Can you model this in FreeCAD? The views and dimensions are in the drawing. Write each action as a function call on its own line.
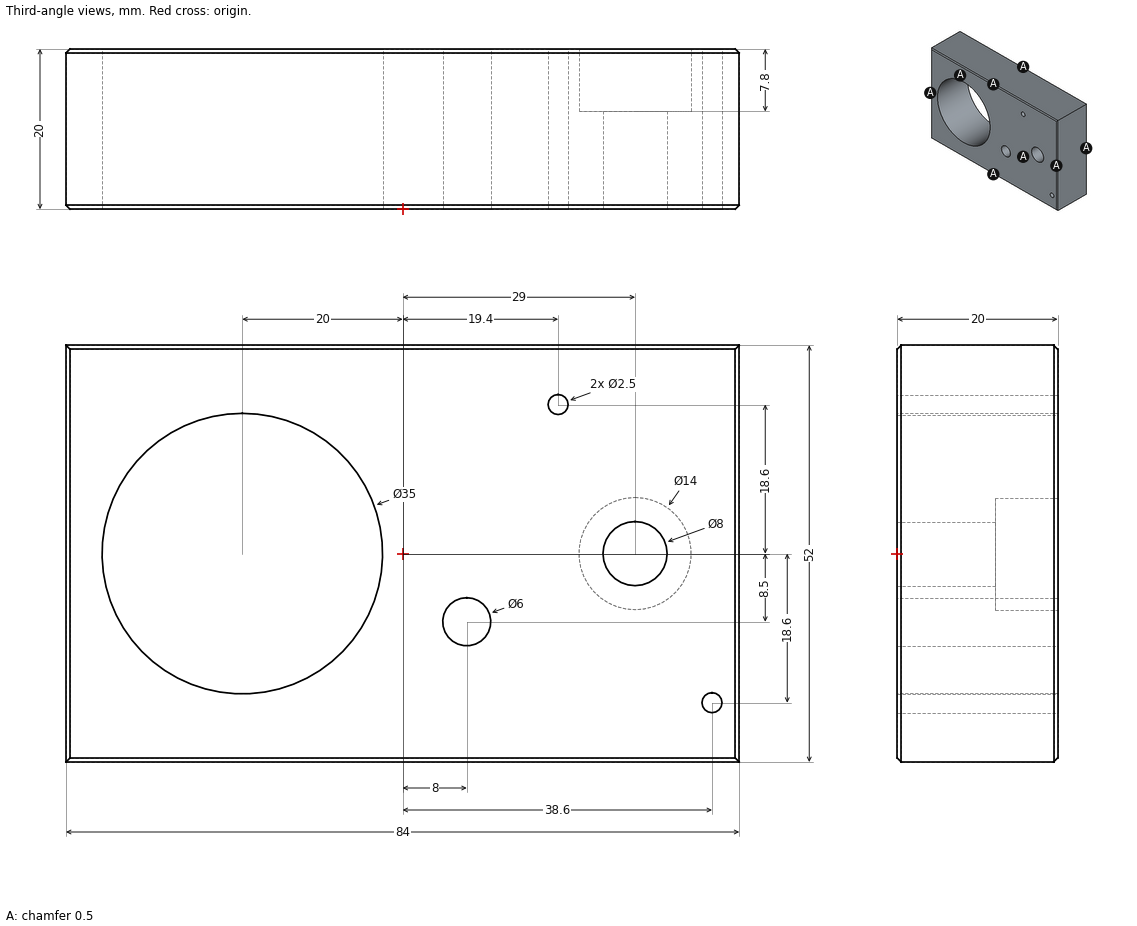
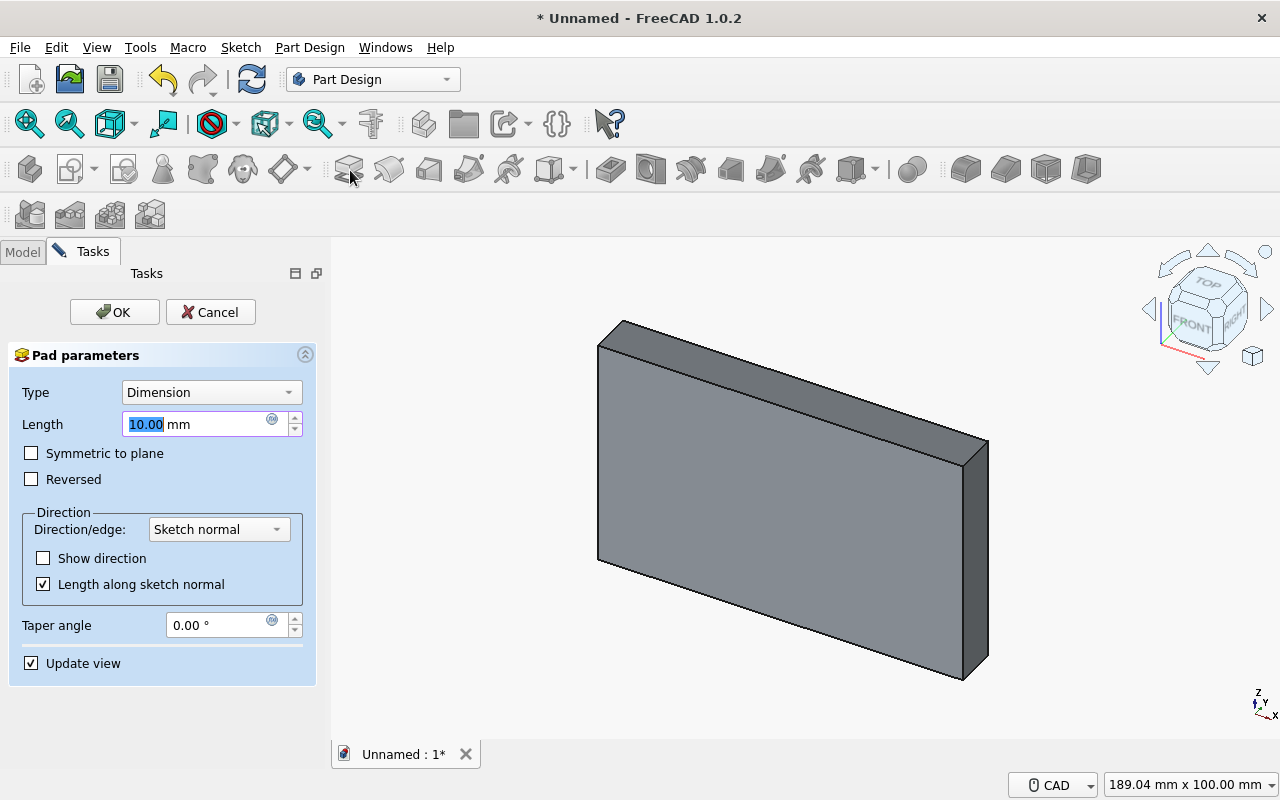
text(20)
key(Tab)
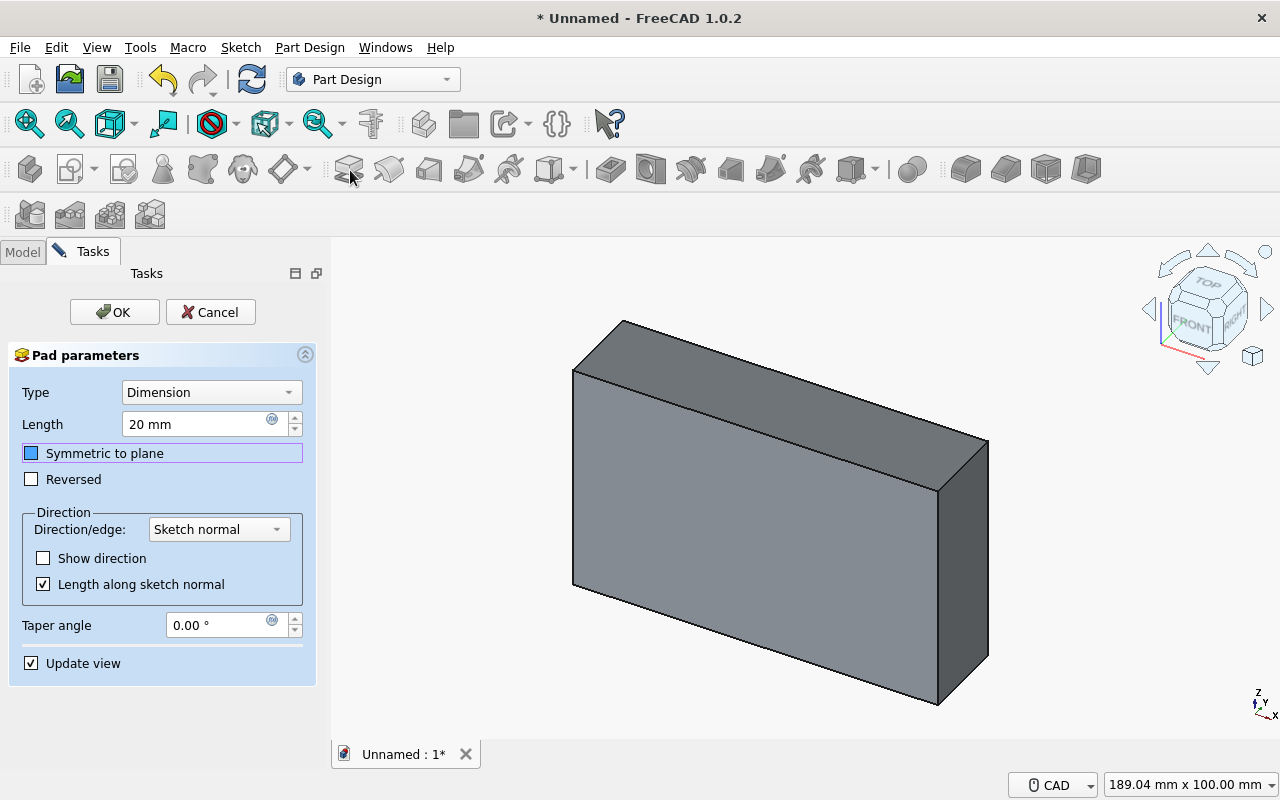
click(30, 479)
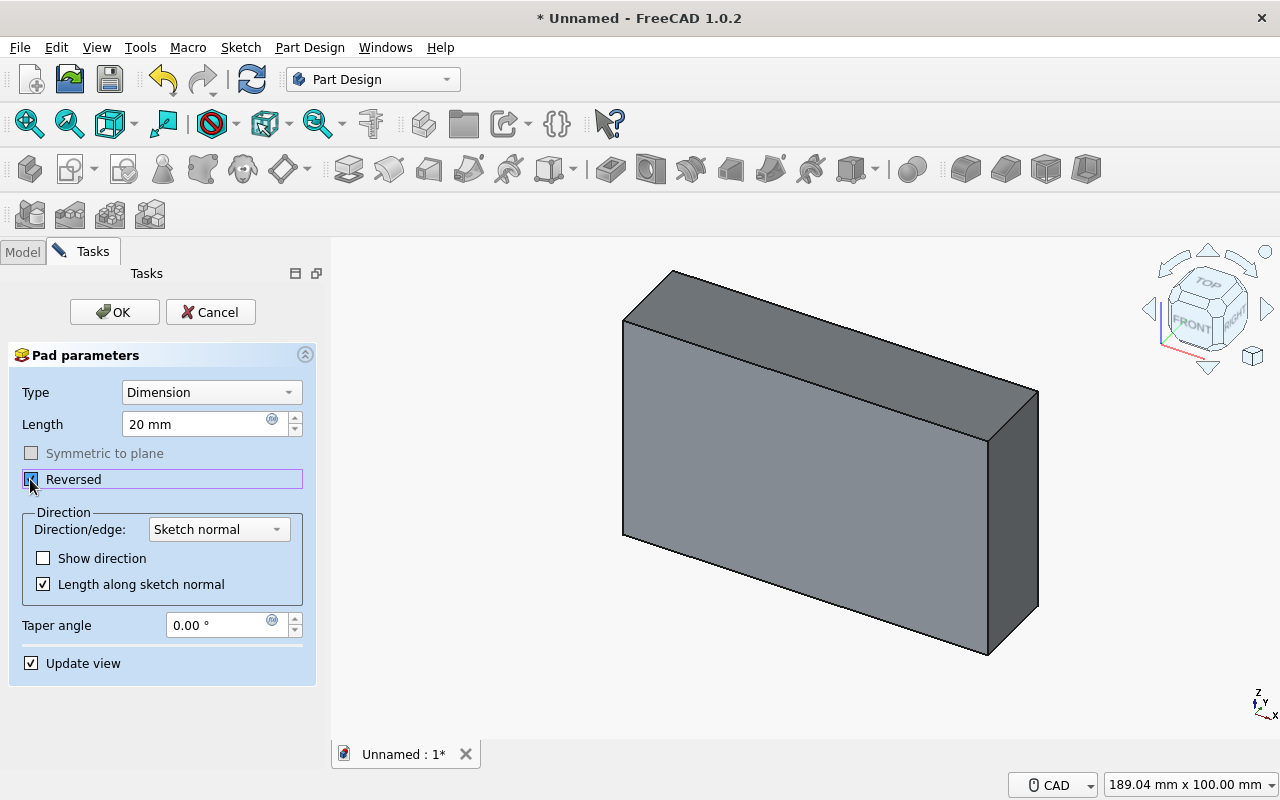
click(115, 312)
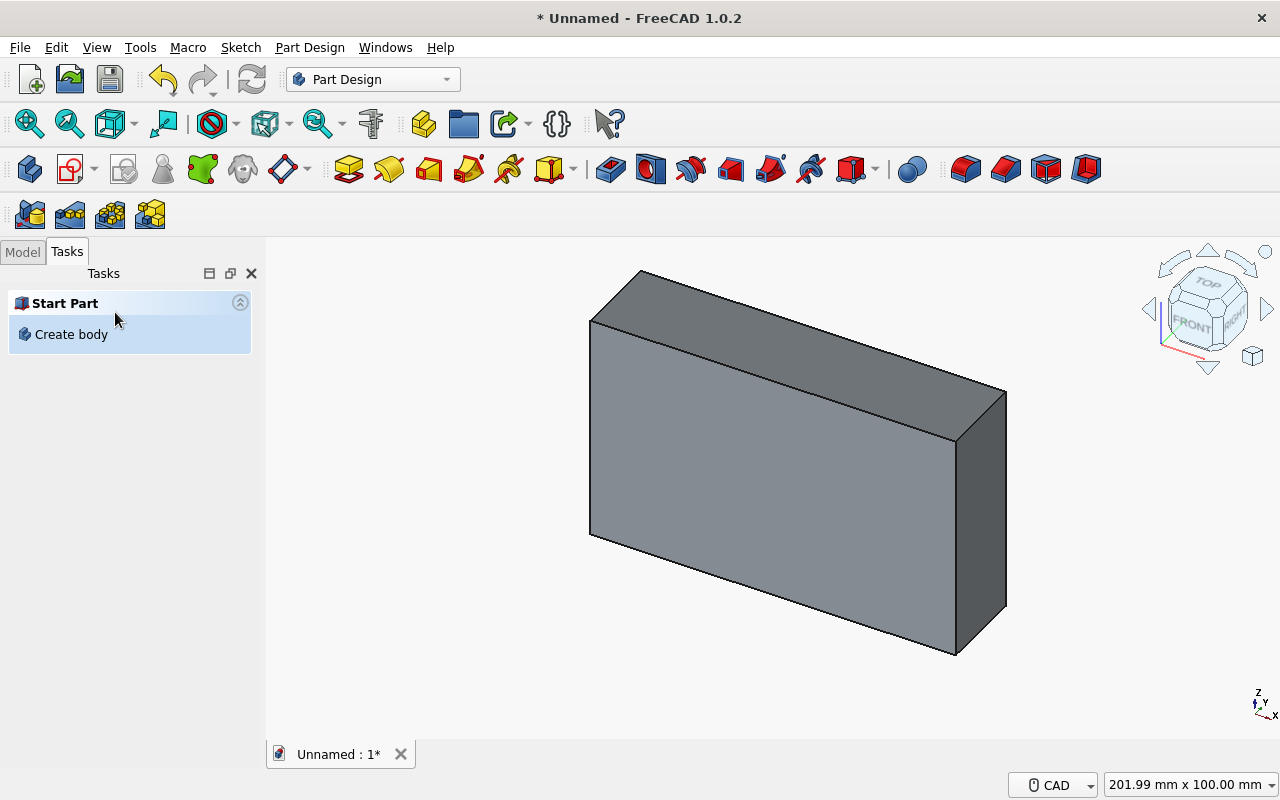
key(4)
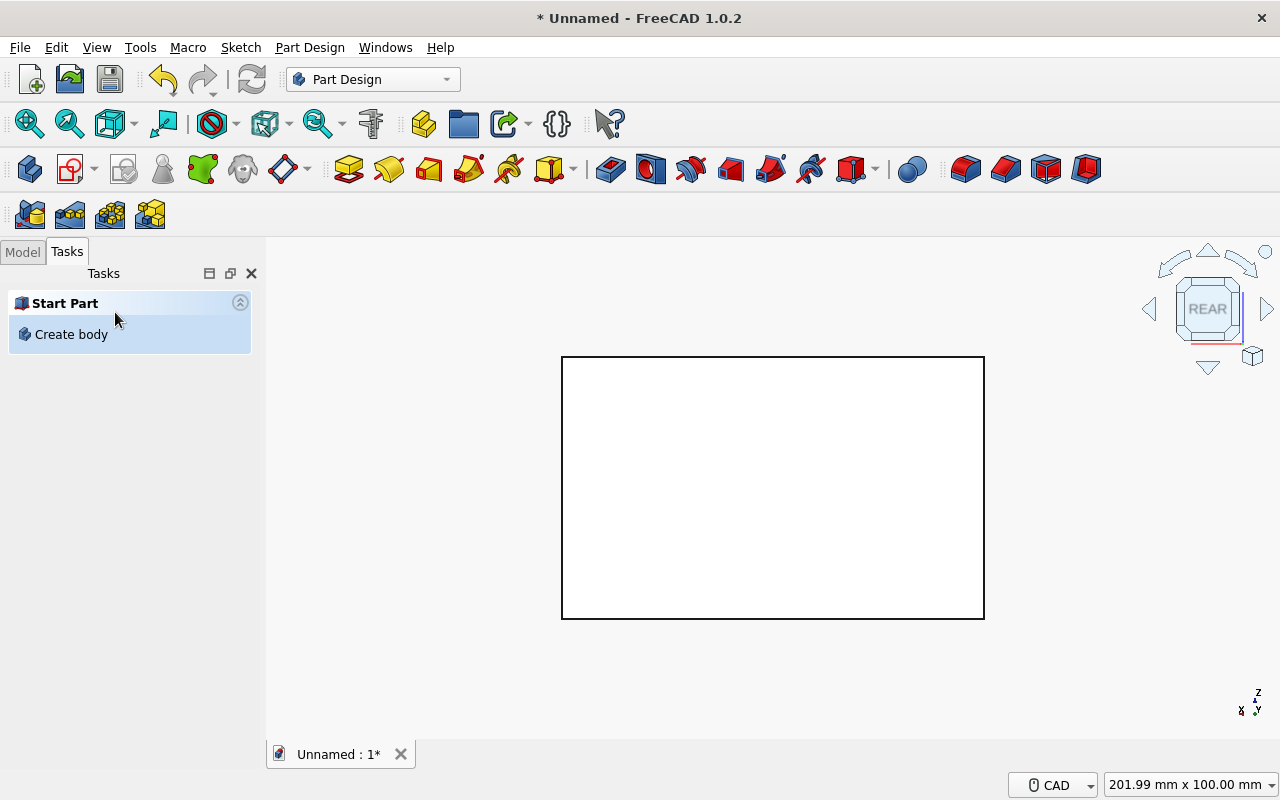
click(713, 487)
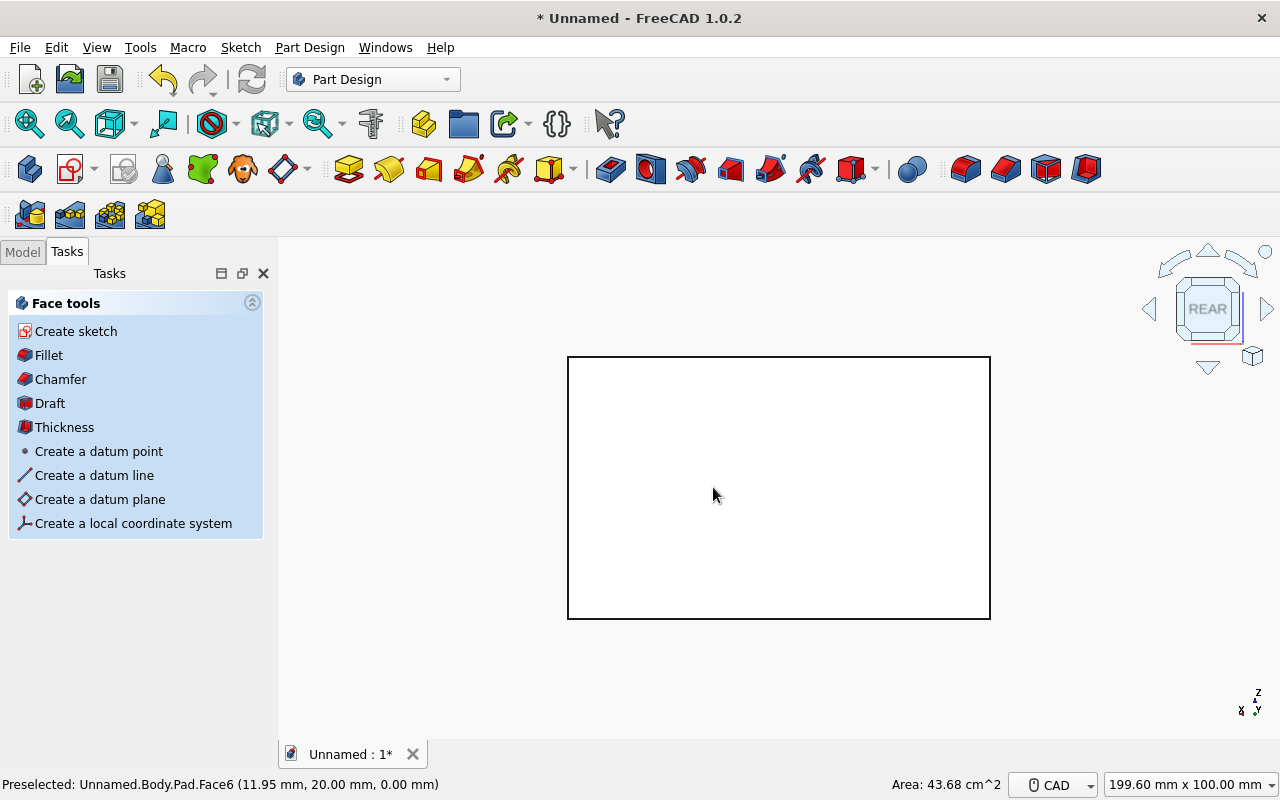
click(70, 170)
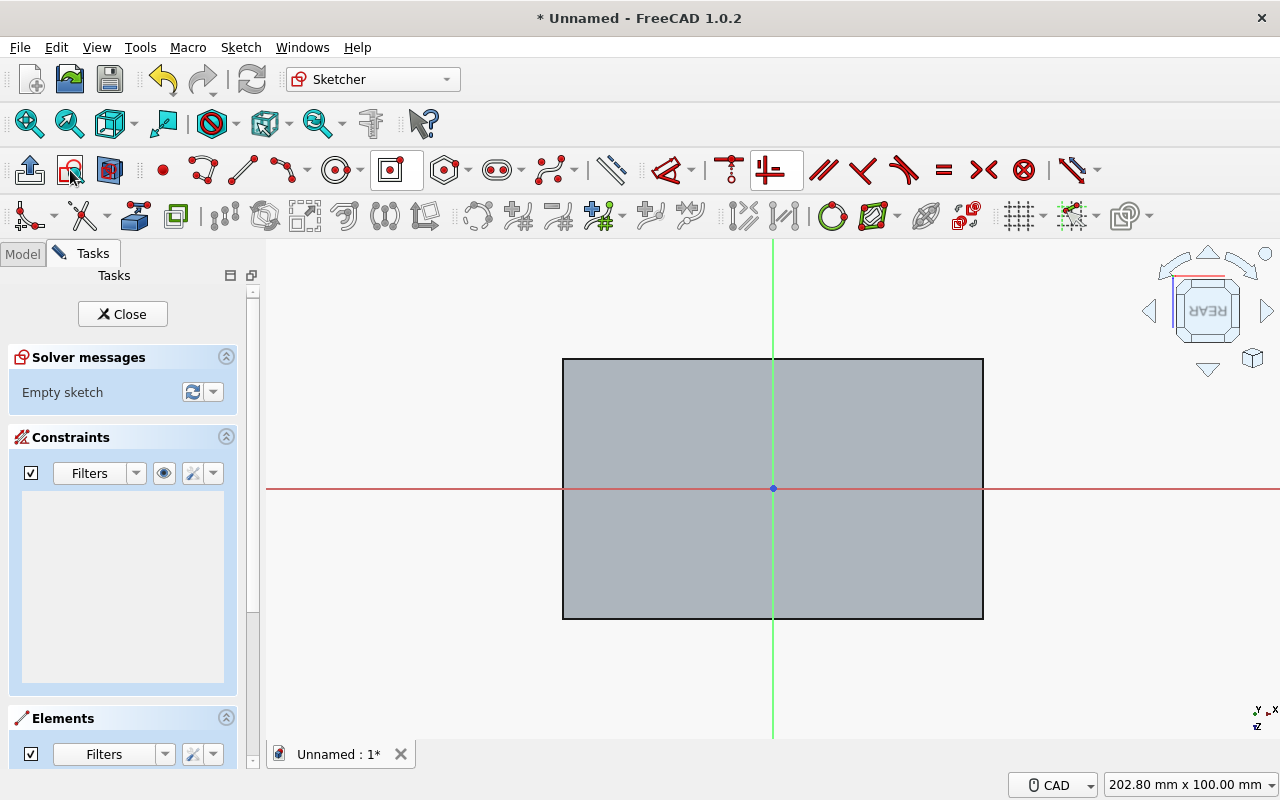
scroll(649, 489, up, 3)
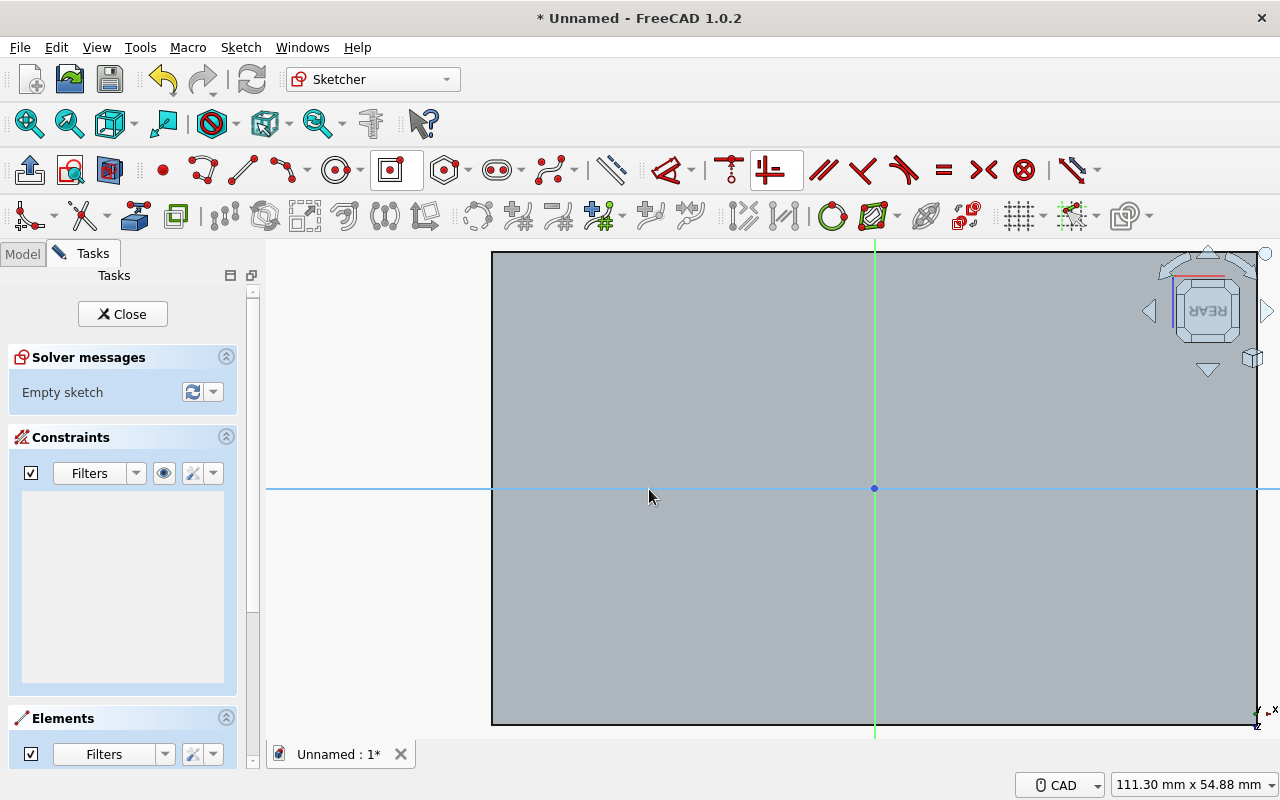
click(336, 170)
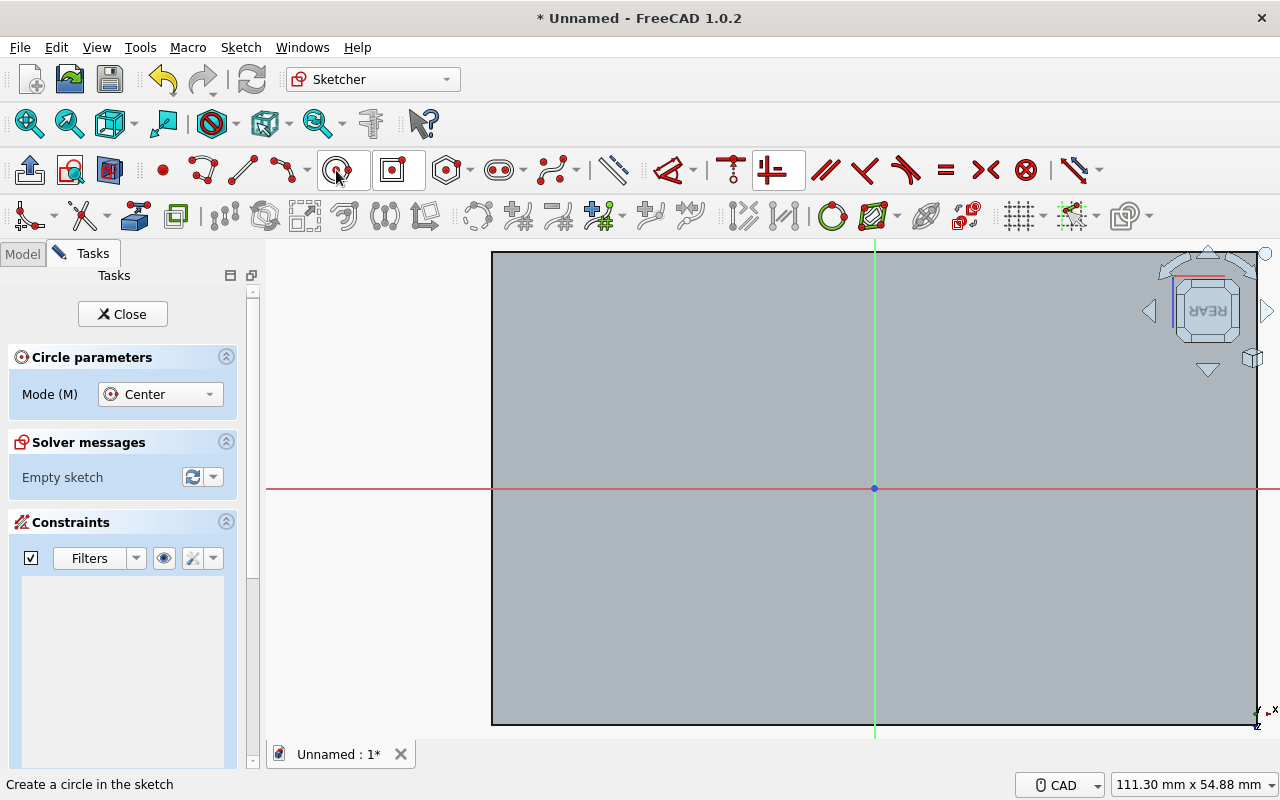
click(692, 489)
move(805, 376)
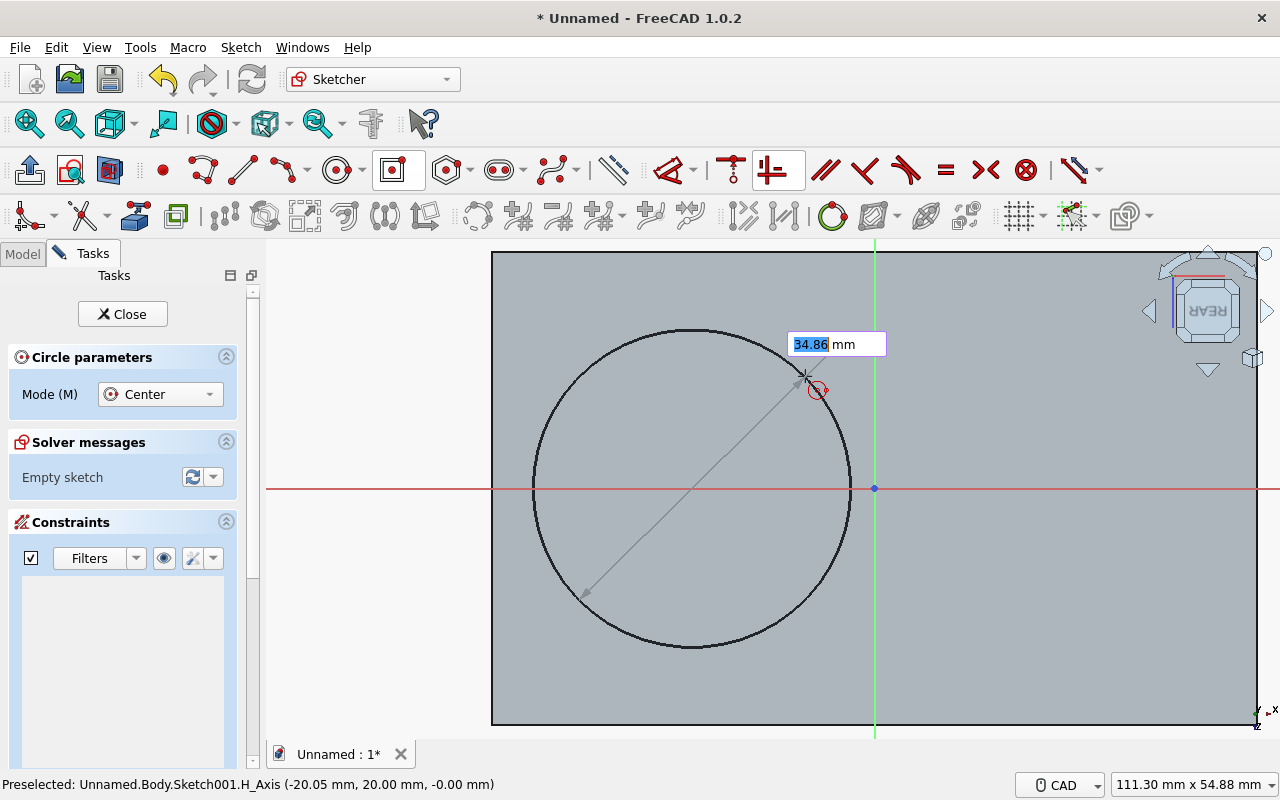
text(35)
key(Return)
key(Escape)